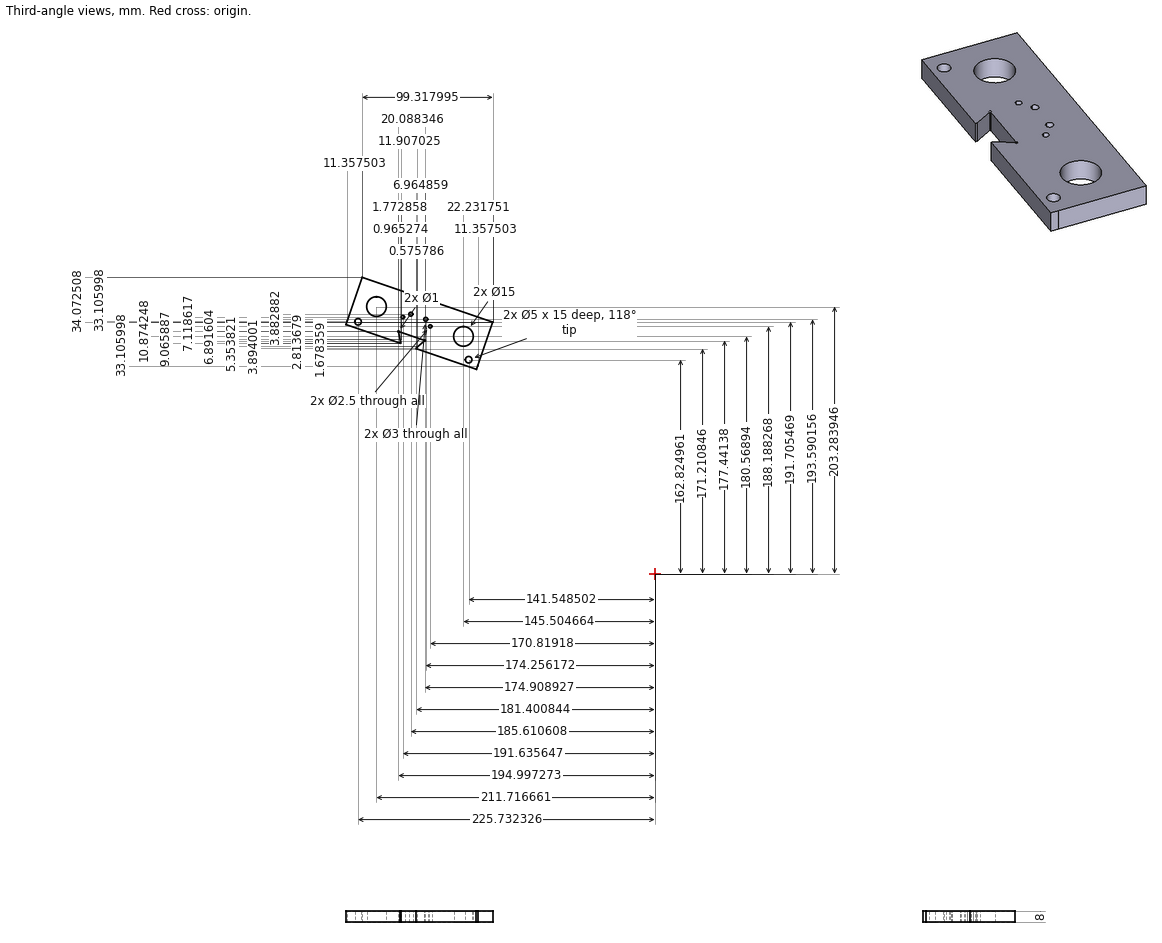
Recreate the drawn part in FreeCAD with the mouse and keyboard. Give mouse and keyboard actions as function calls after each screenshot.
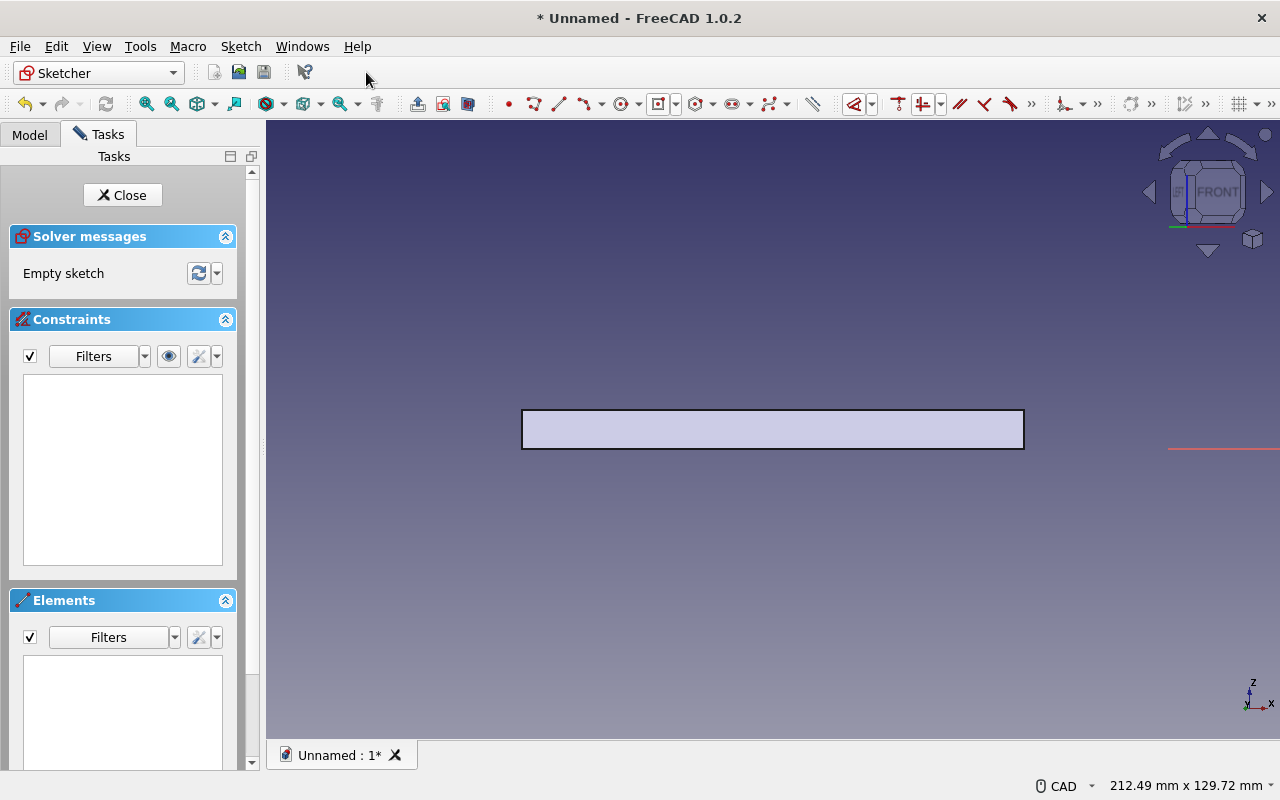
key(g)
key(r)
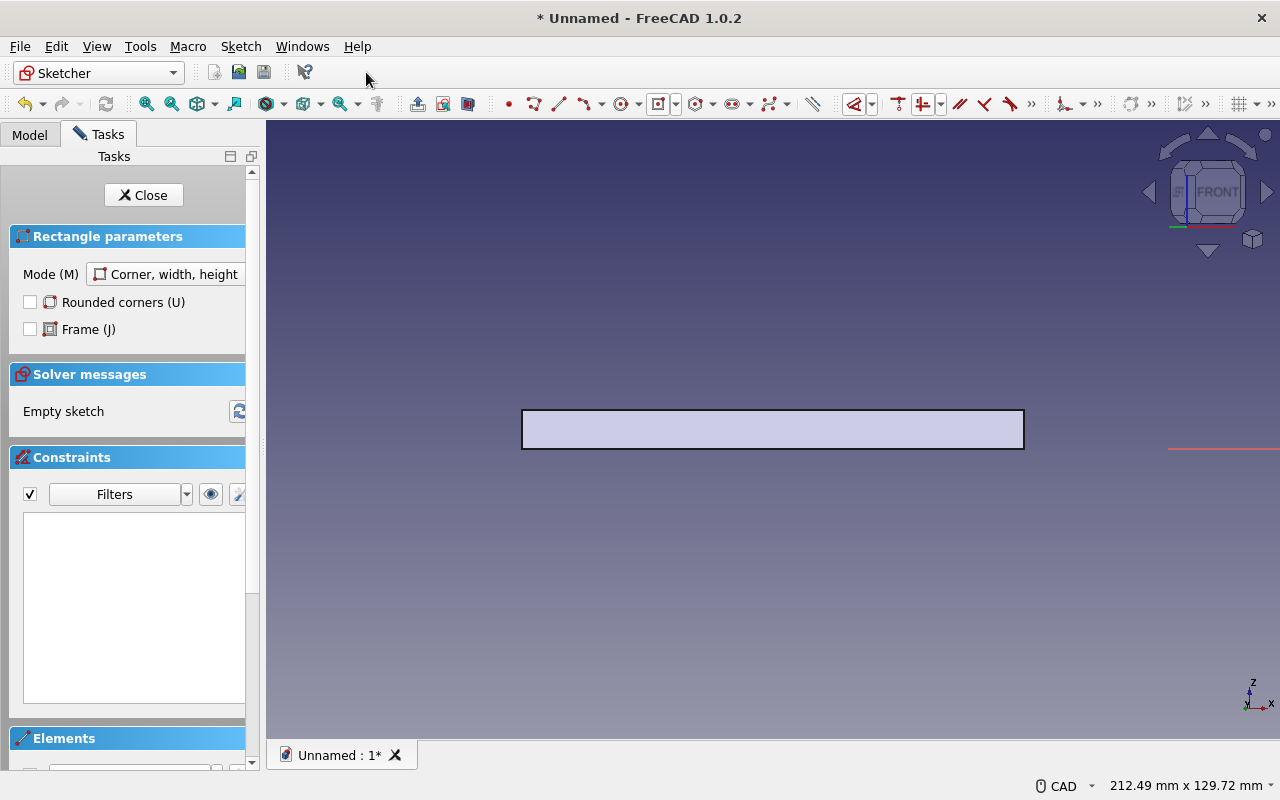
click(522, 410)
click(1024, 449)
key(Escape)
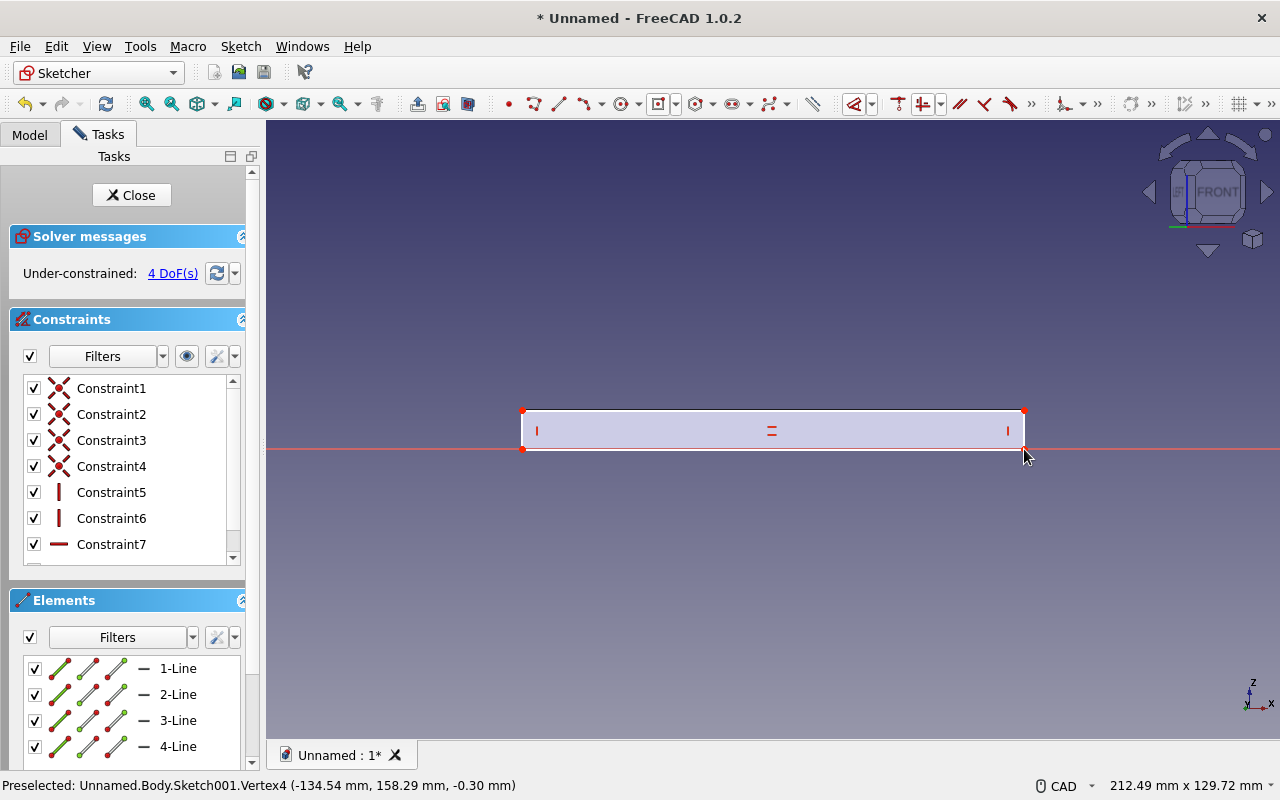
click(522, 450)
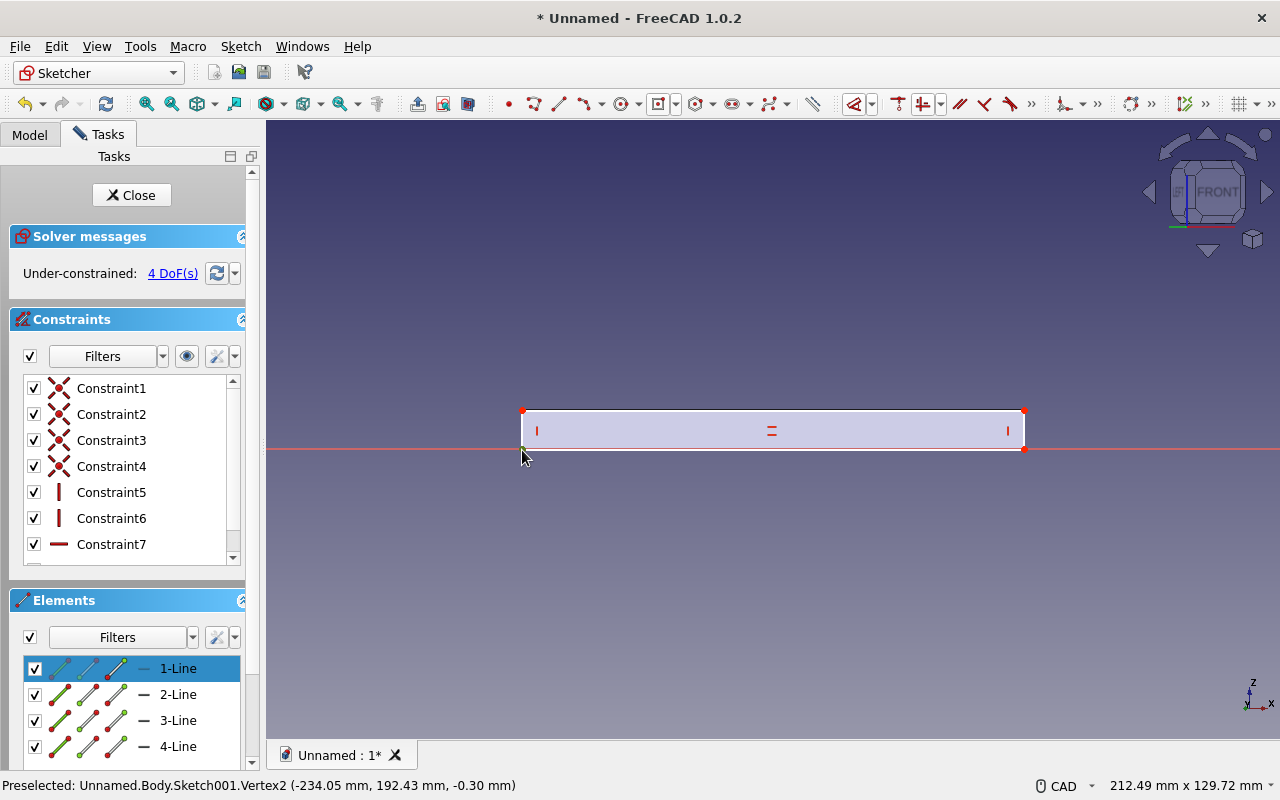
click(353, 449)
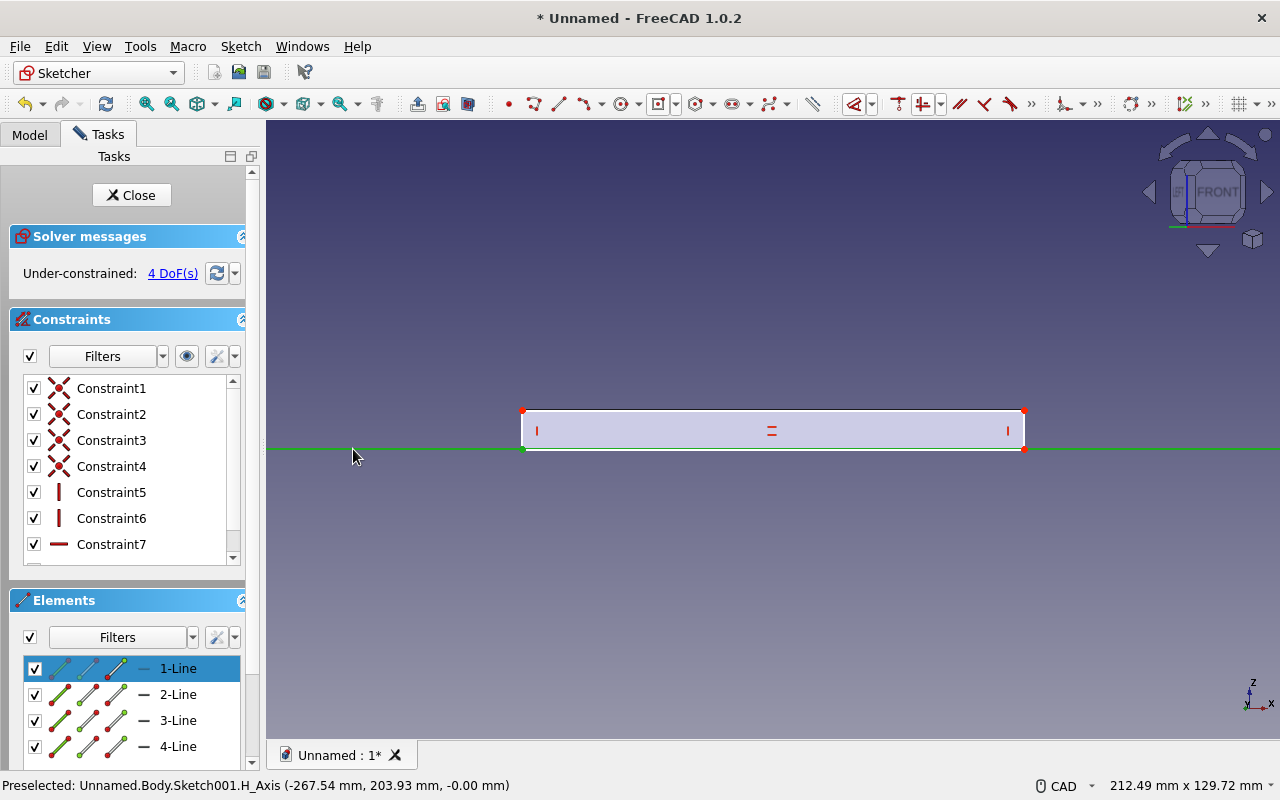
click(898, 104)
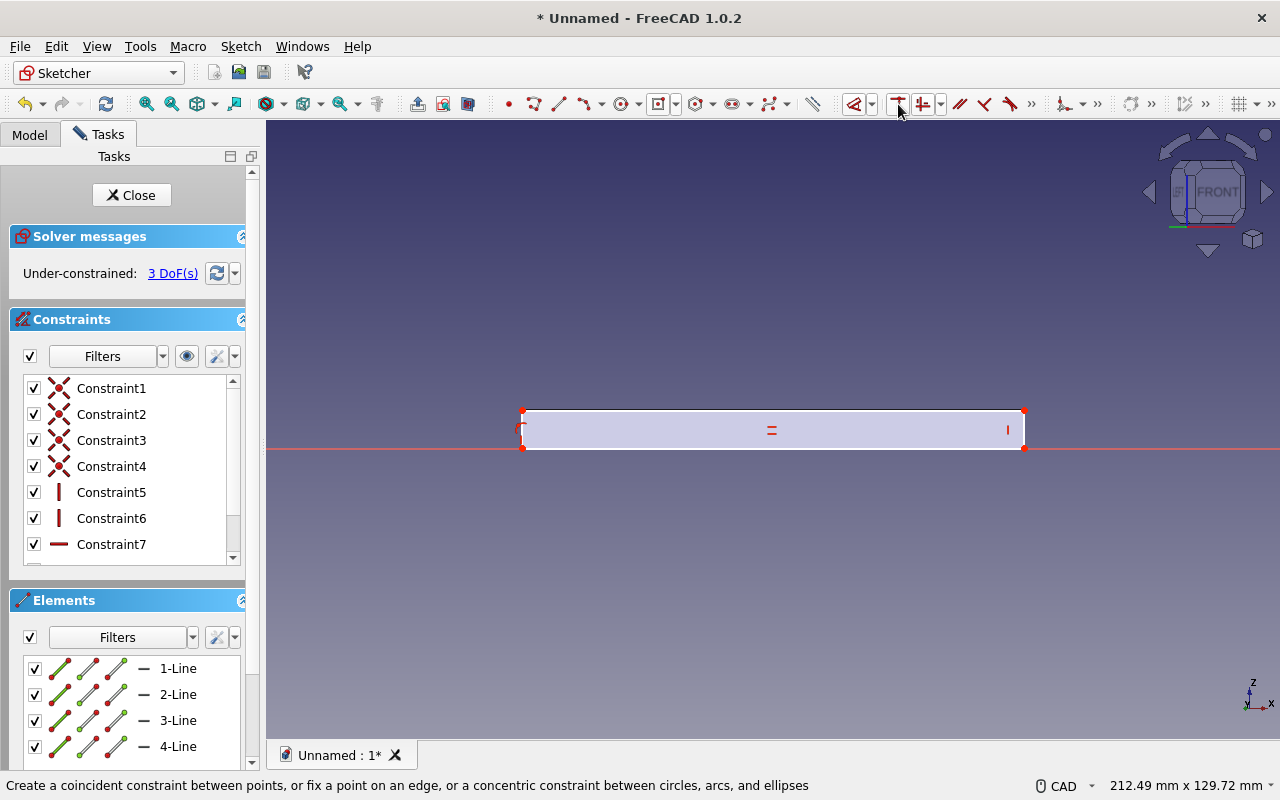
scroll(522, 422, up, 2)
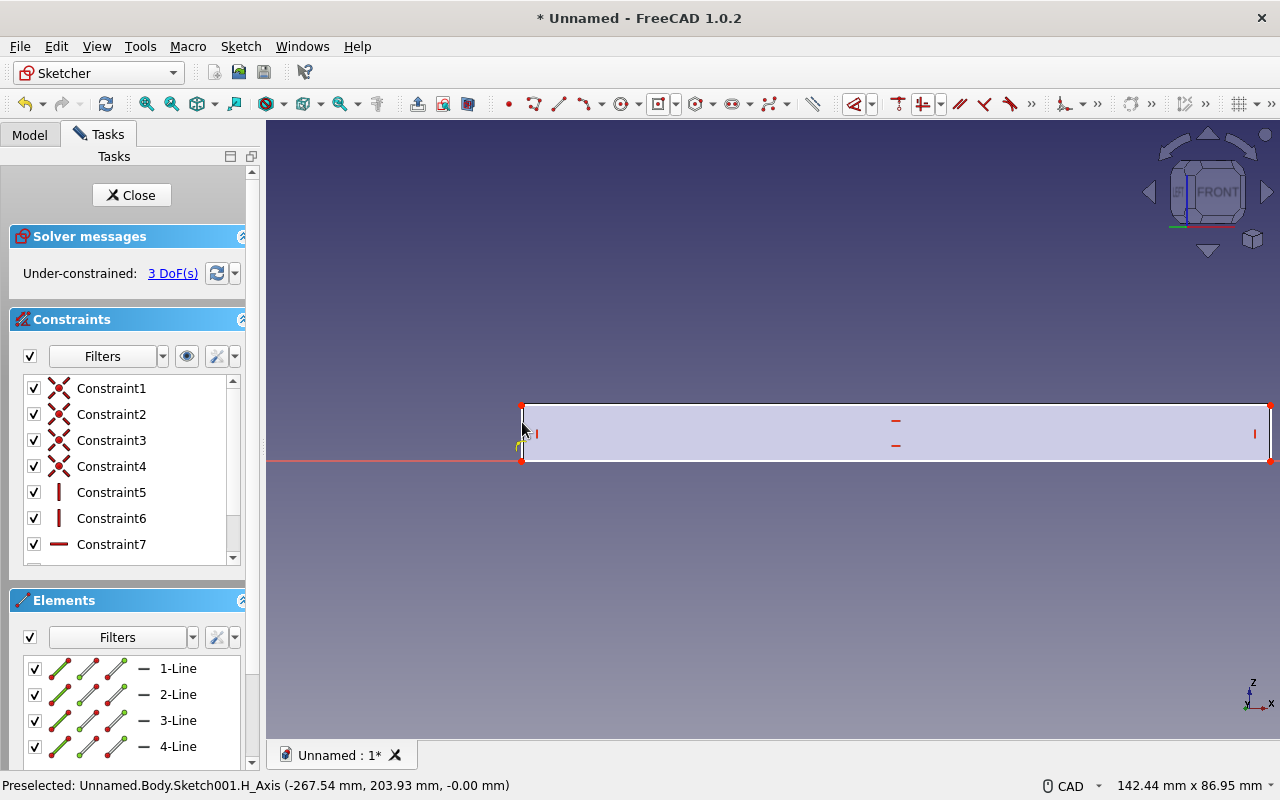
click(522, 422)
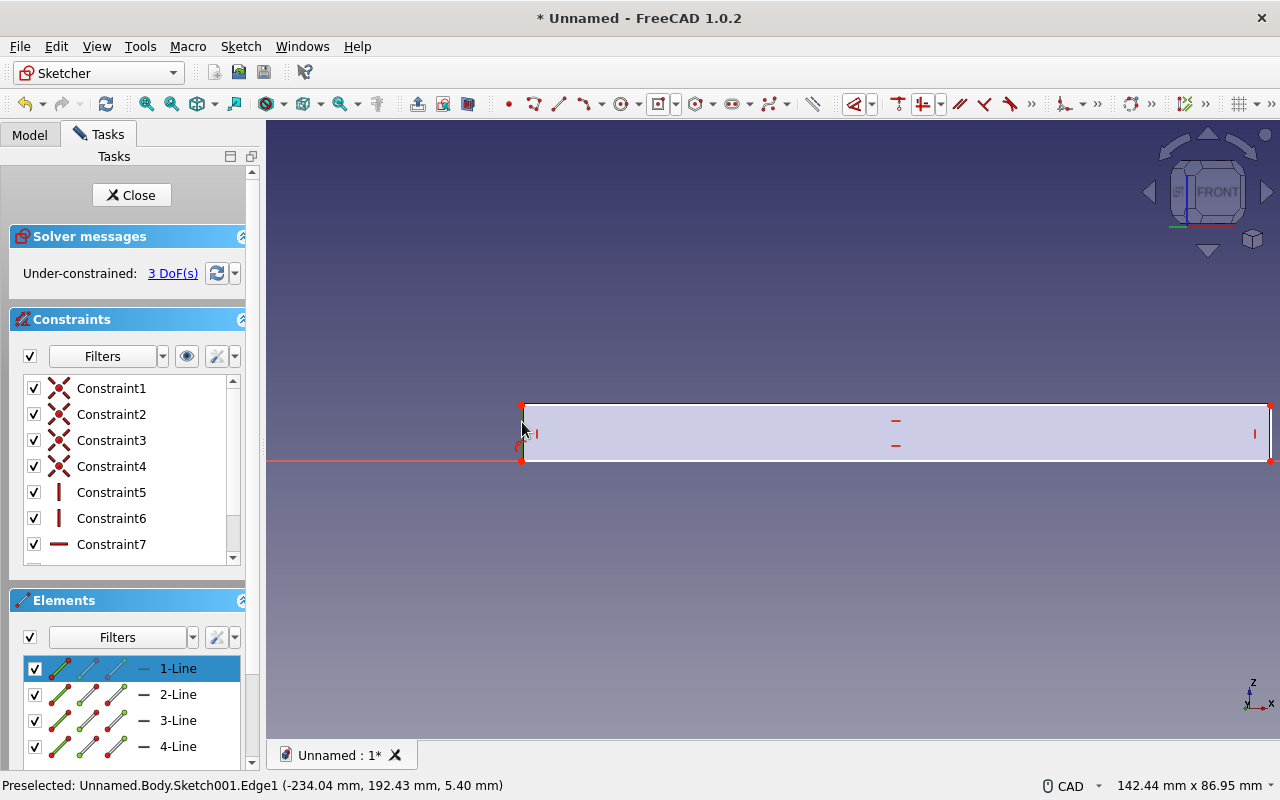
click(872, 104)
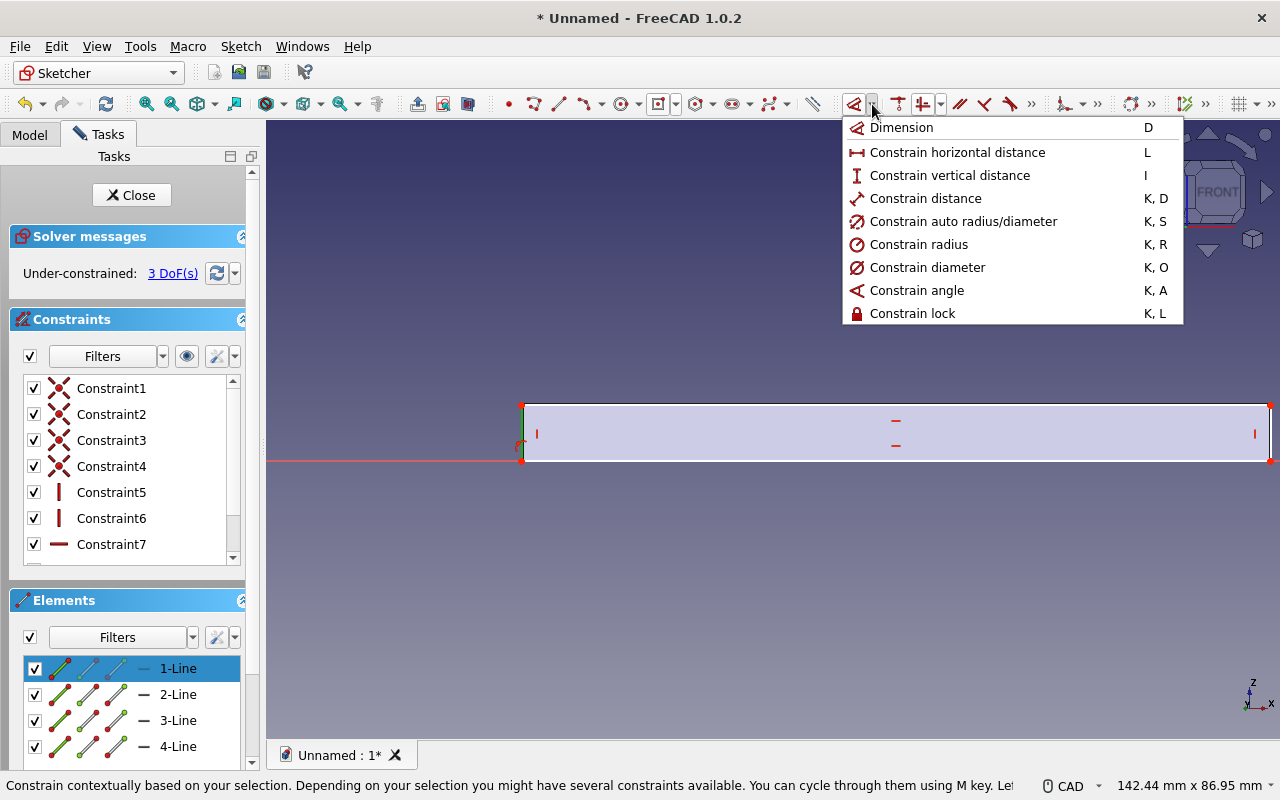
click(1013, 176)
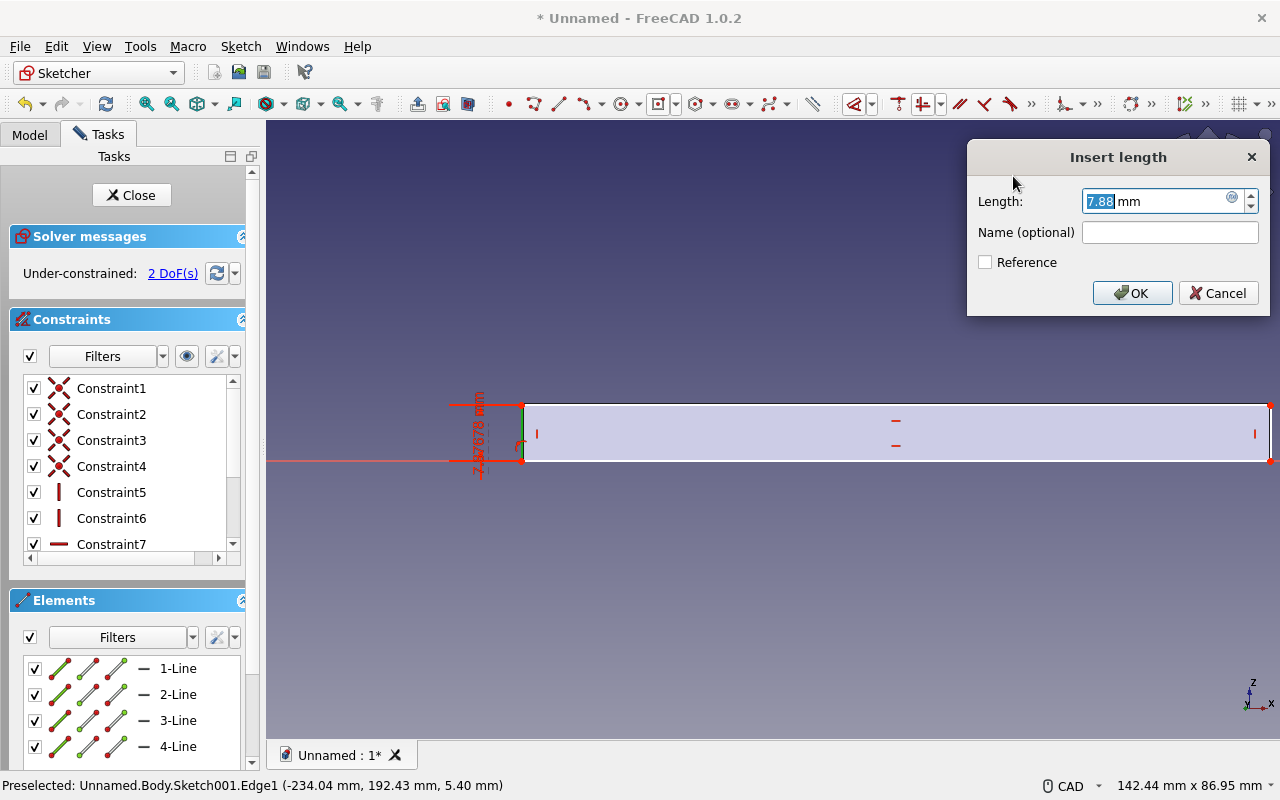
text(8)
key(Return)